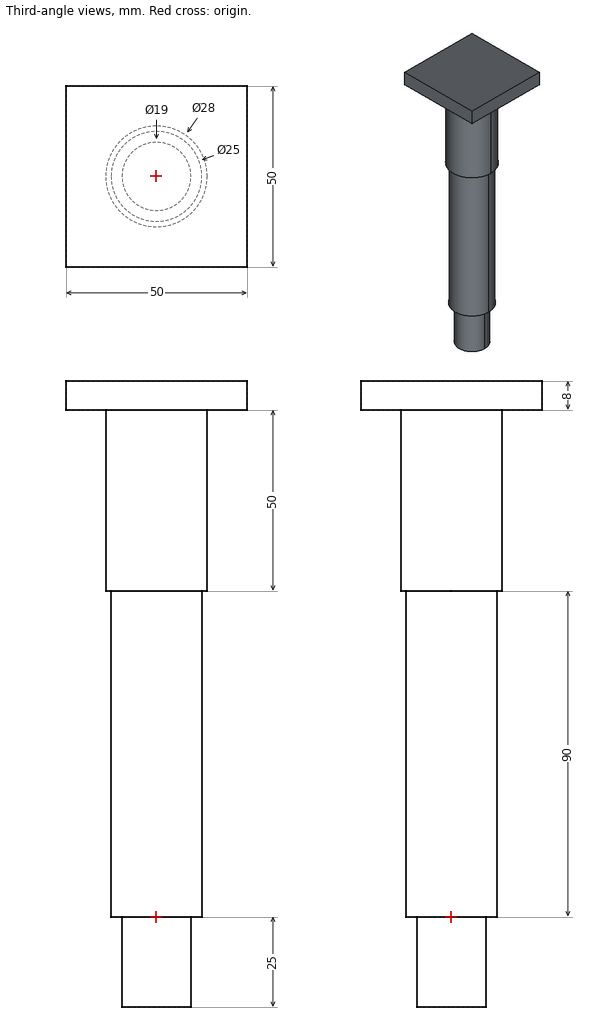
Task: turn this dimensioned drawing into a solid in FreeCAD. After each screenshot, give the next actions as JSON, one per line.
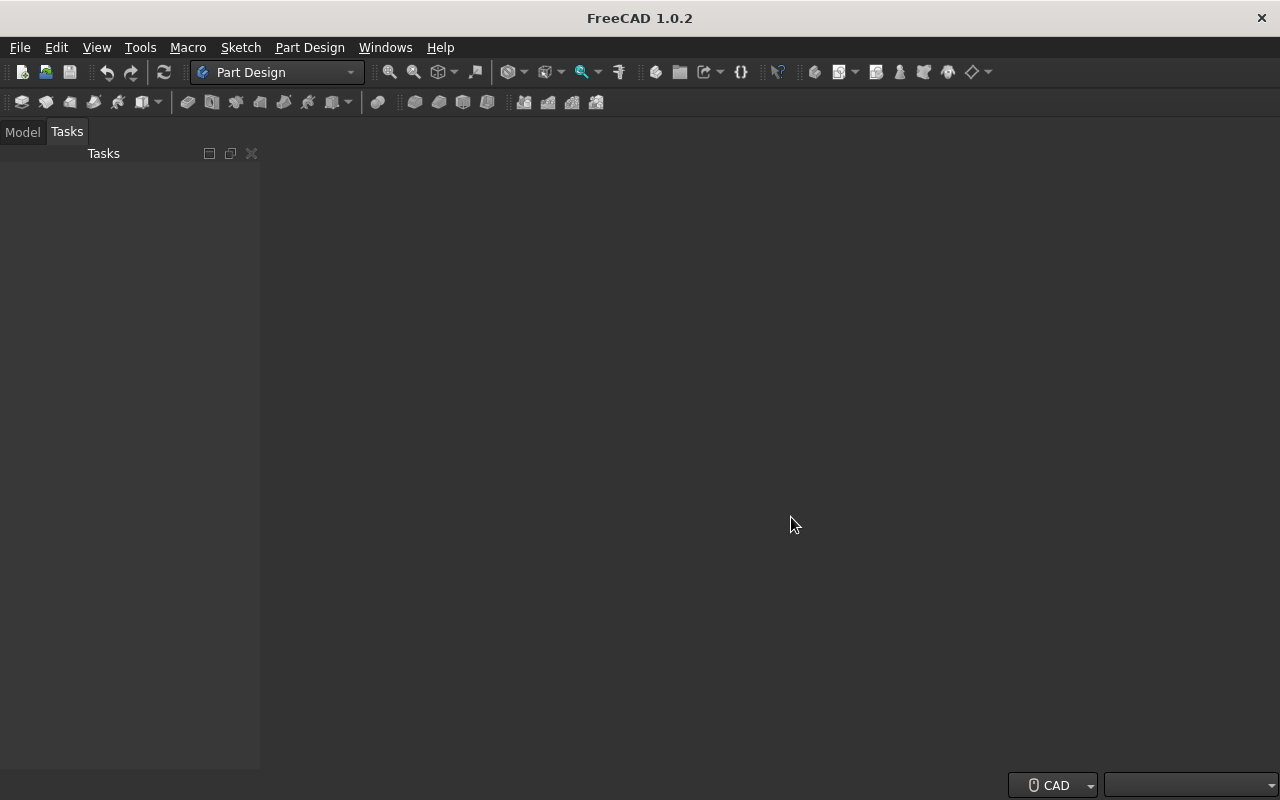
{"action": "left_click", "coordinate": [22, 72]}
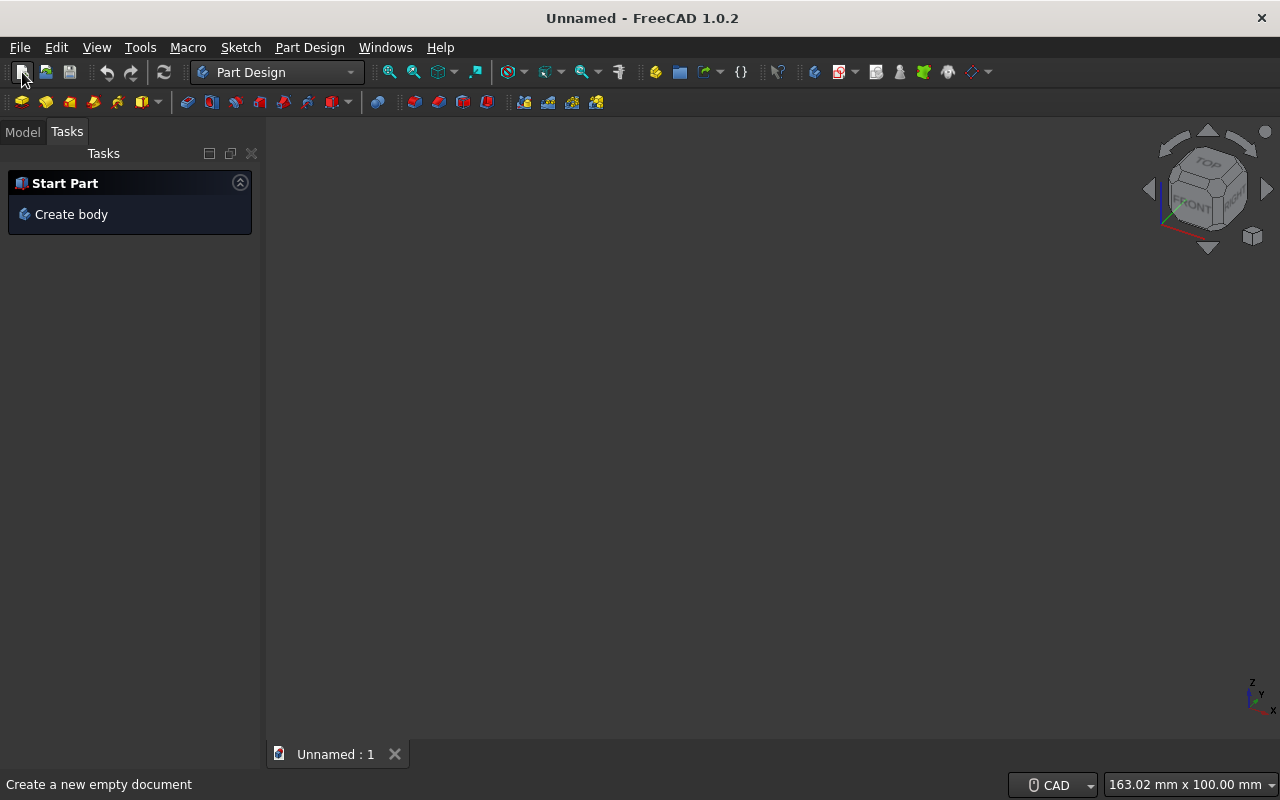
{"action": "left_click", "coordinate": [840, 72]}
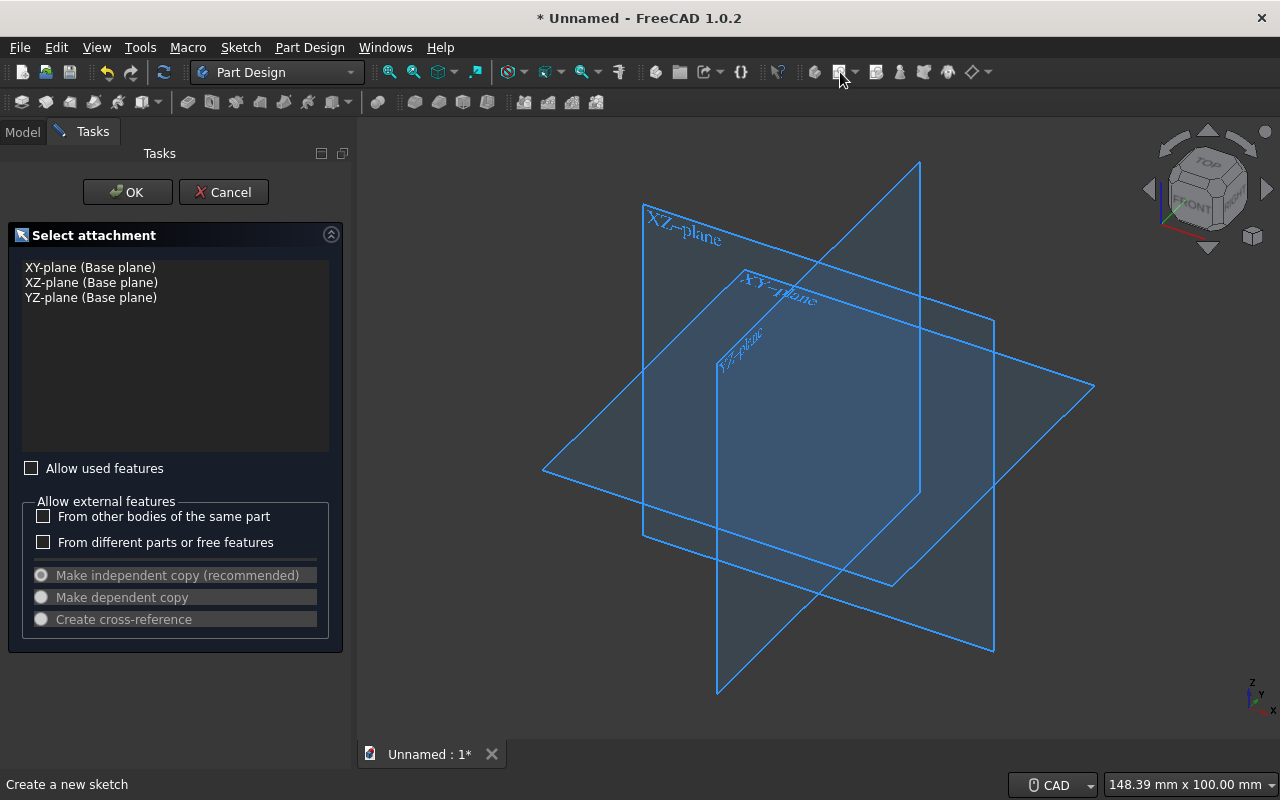
{"action": "left_click", "coordinate": [82, 268]}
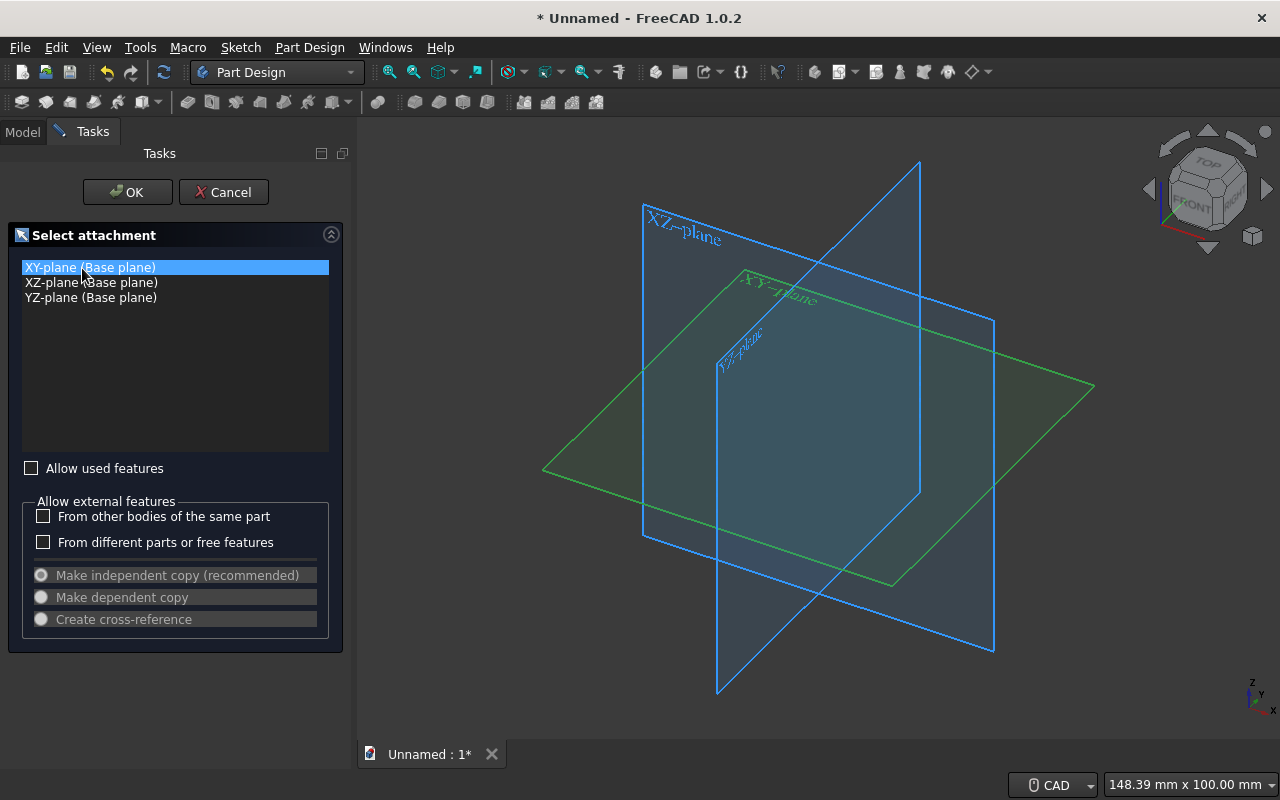
{"action": "left_click", "coordinate": [128, 192]}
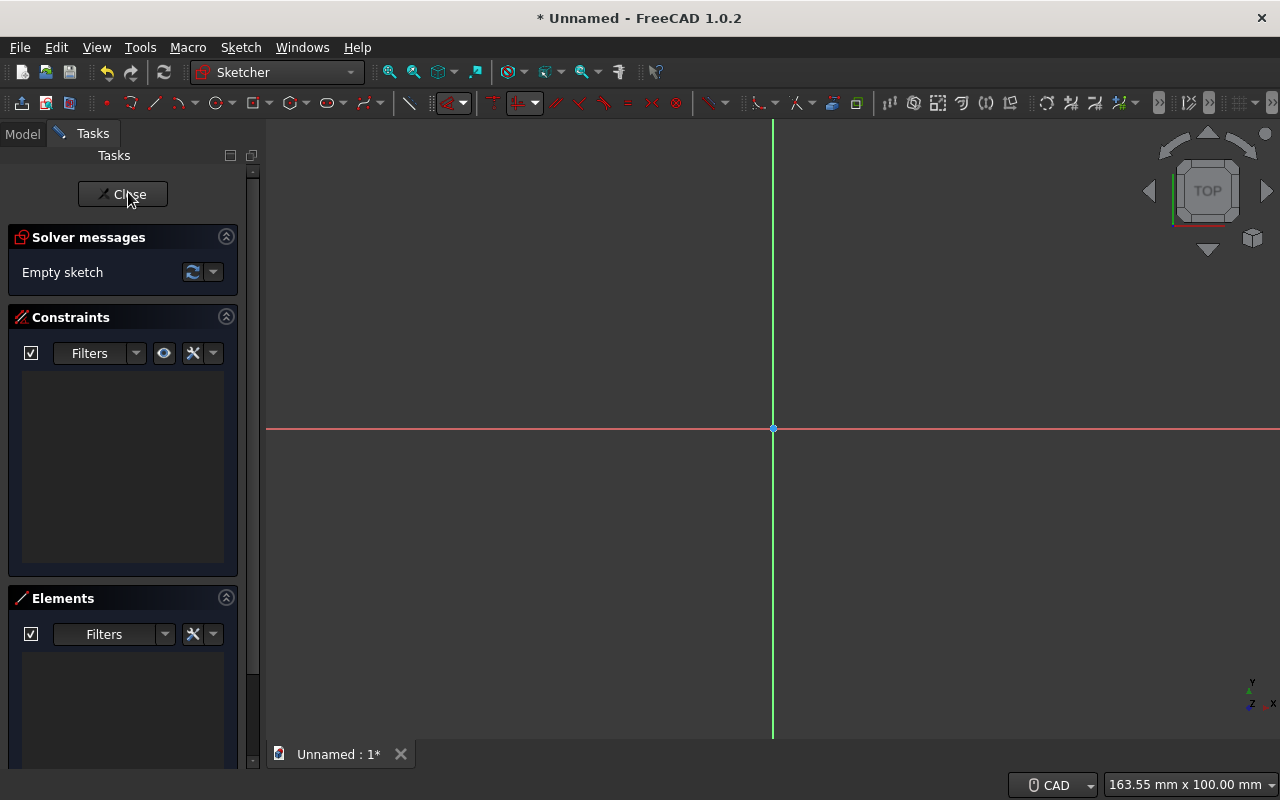
{"action": "scroll", "coordinate": [813, 429], "scroll_direction": "up", "scroll_amount": 5}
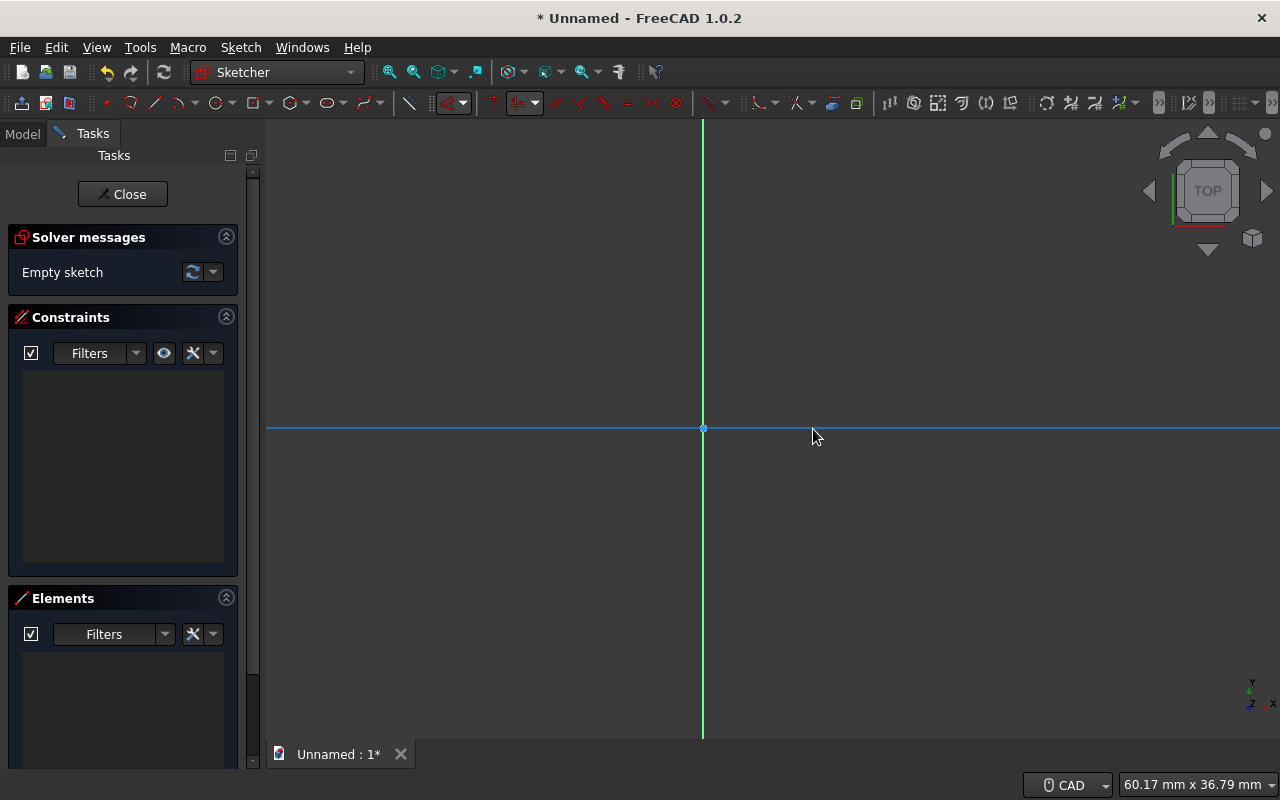
{"action": "key", "text": "g c"}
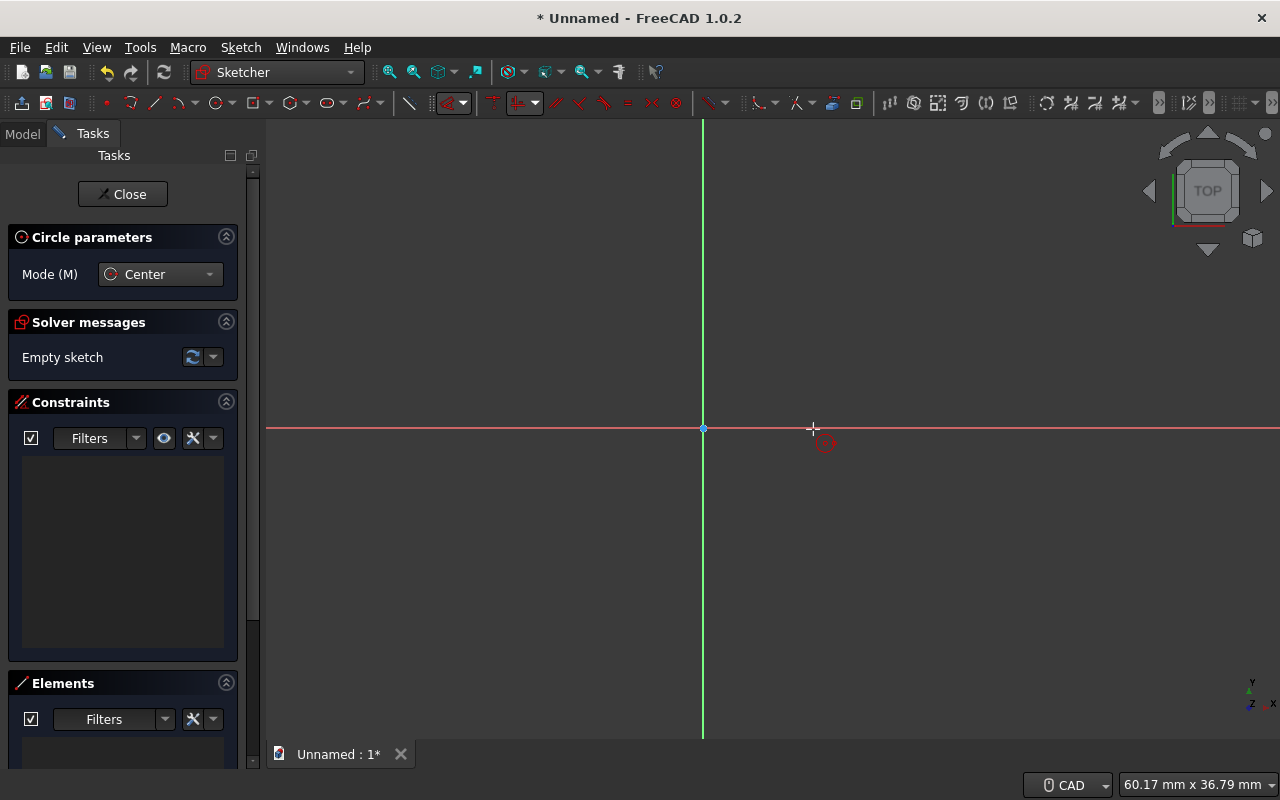
{"action": "left_click", "coordinate": [703, 428]}
{"action": "left_click", "coordinate": [852, 279]}
{"action": "key", "text": "Escape"}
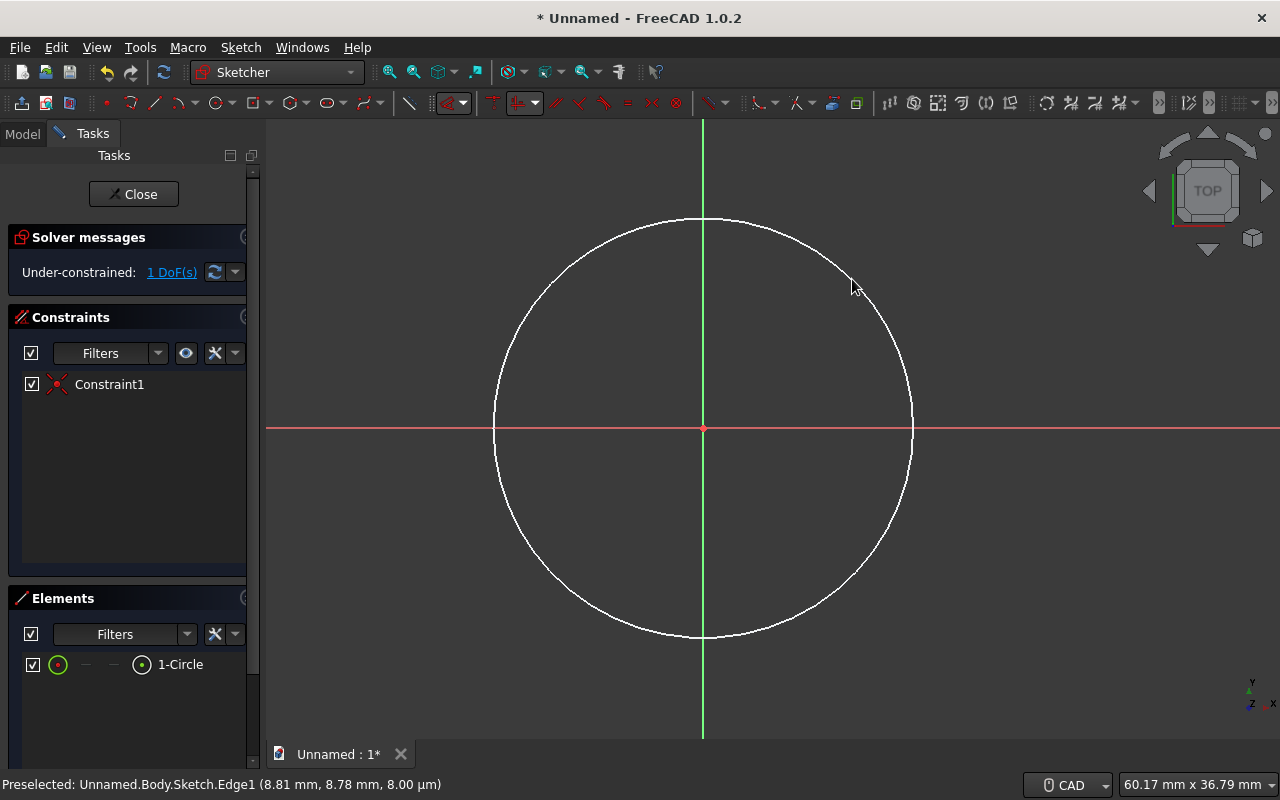
{"action": "key", "text": "d"}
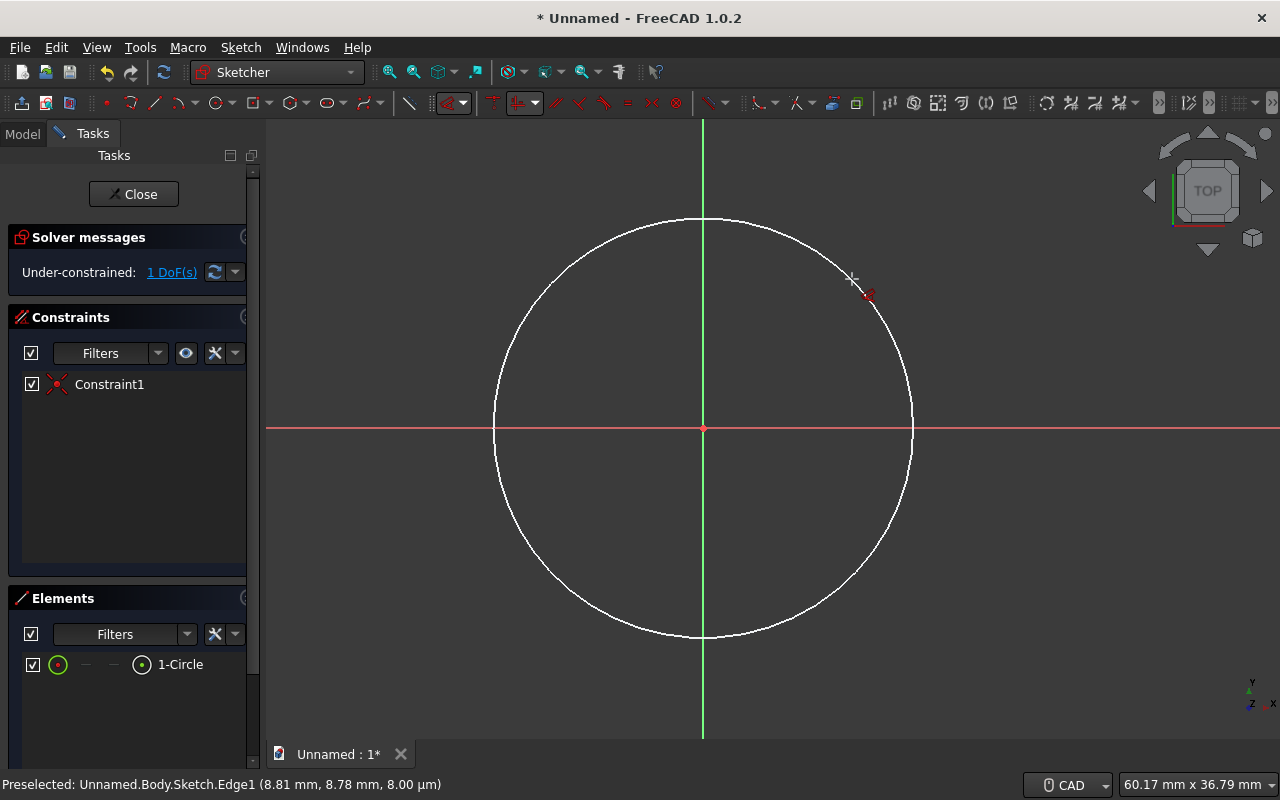
{"action": "left_click", "coordinate": [851, 279]}
{"action": "left_click", "coordinate": [874, 256]}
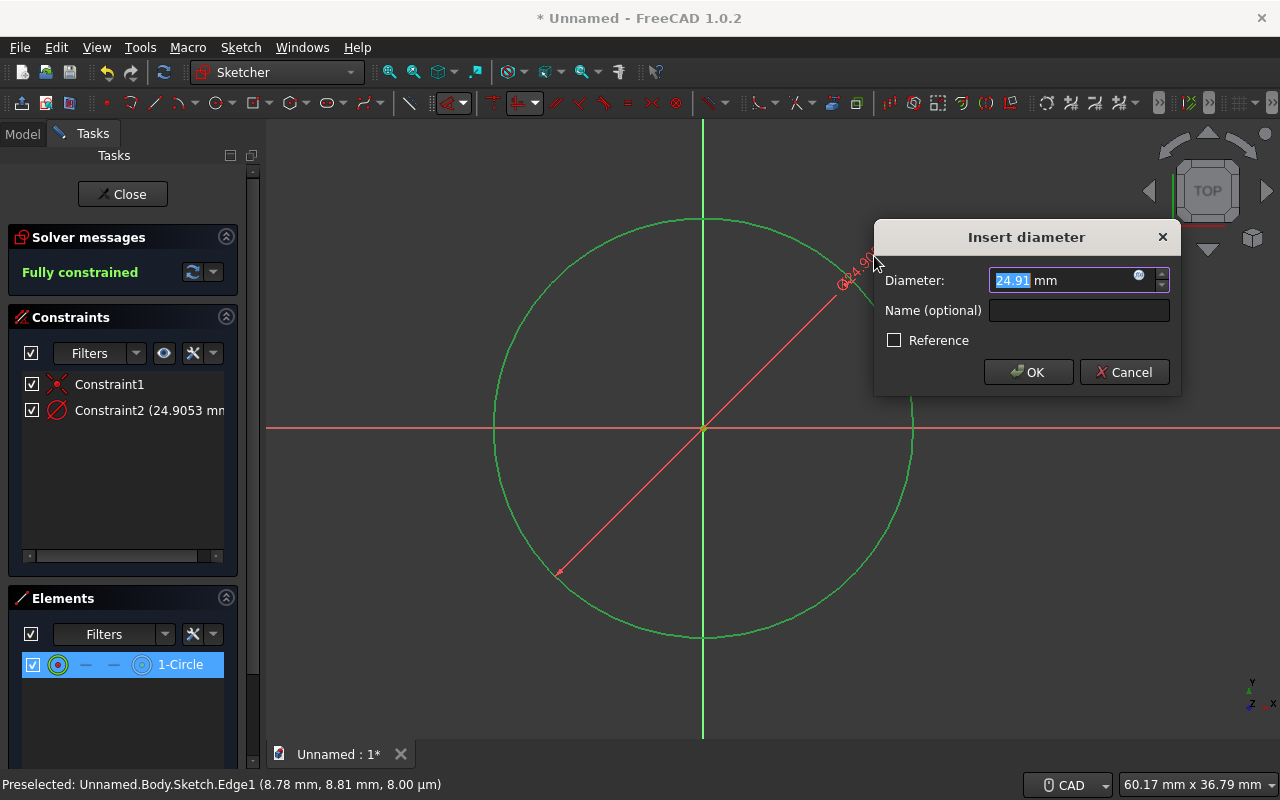
{"action": "type", "text": "25"}
{"action": "key", "text": "Return"}
{"action": "key", "text": "Escape"}